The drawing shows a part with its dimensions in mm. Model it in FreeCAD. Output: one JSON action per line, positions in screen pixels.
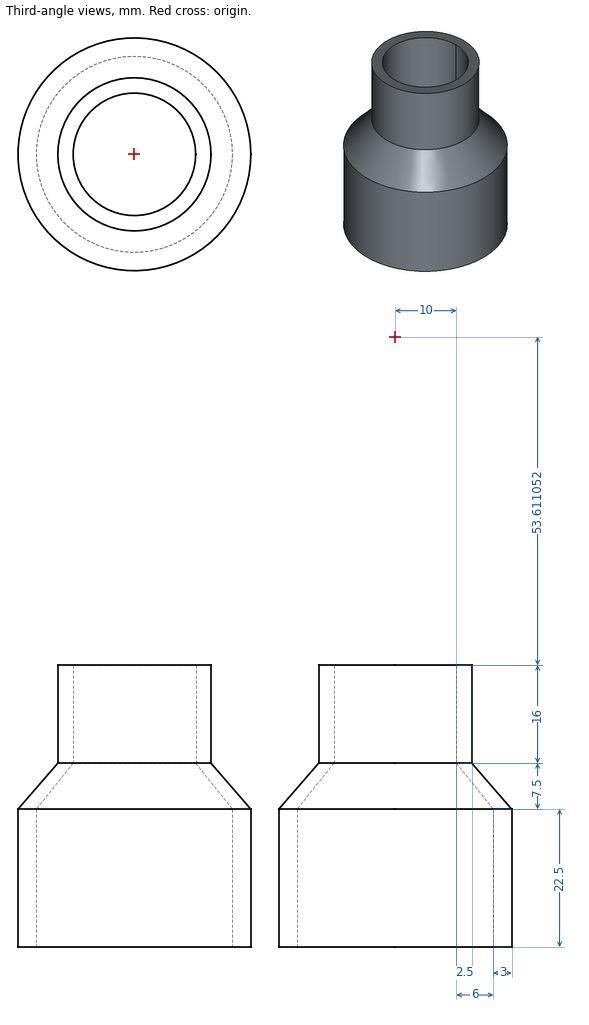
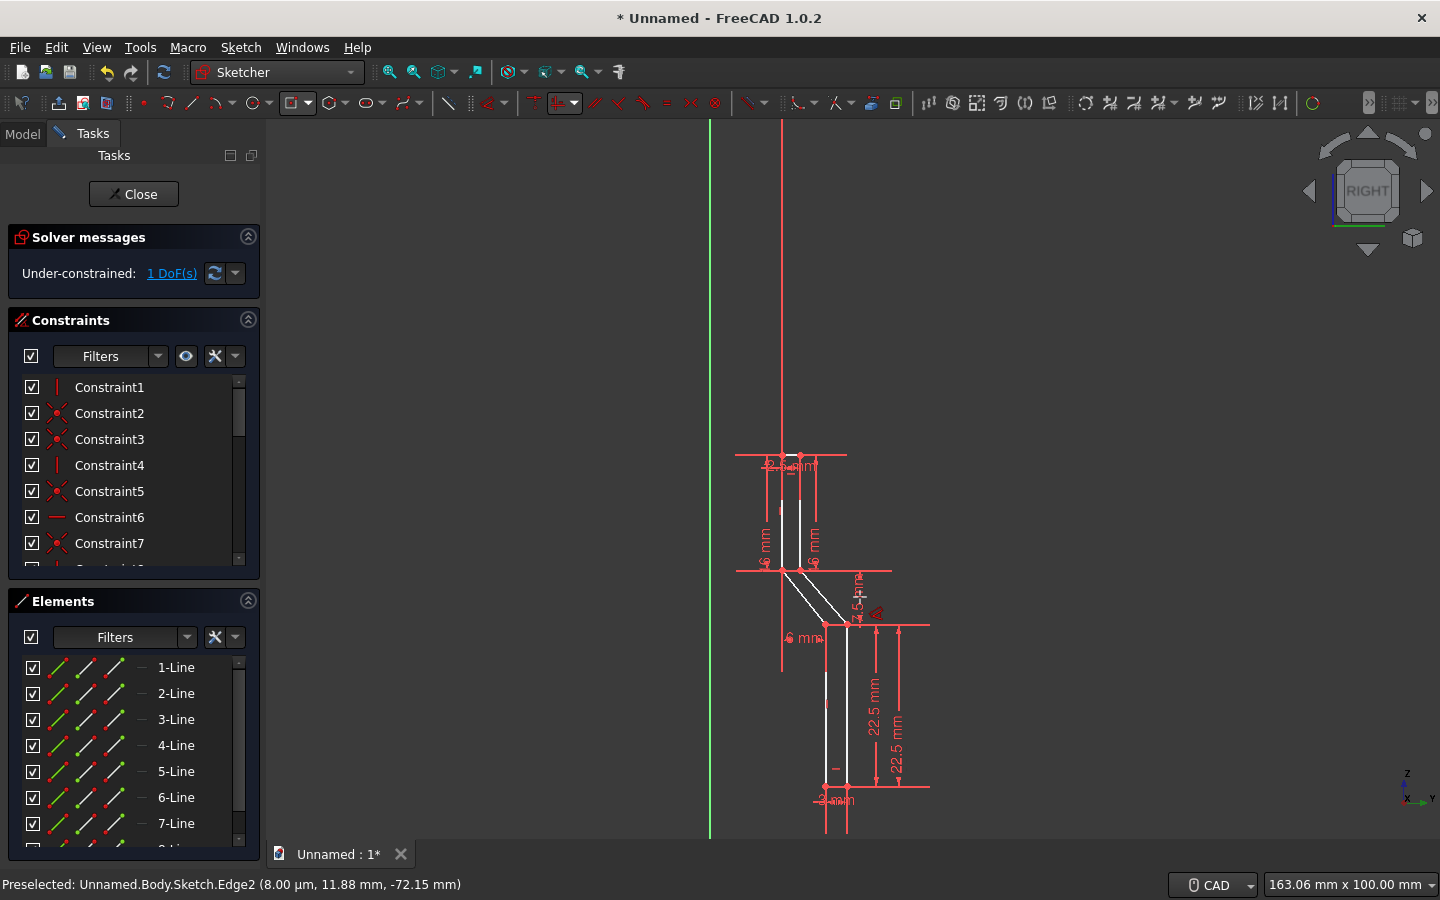
{"action": "left_click", "coordinate": [782, 455]}
{"action": "left_click", "coordinate": [676, 301]}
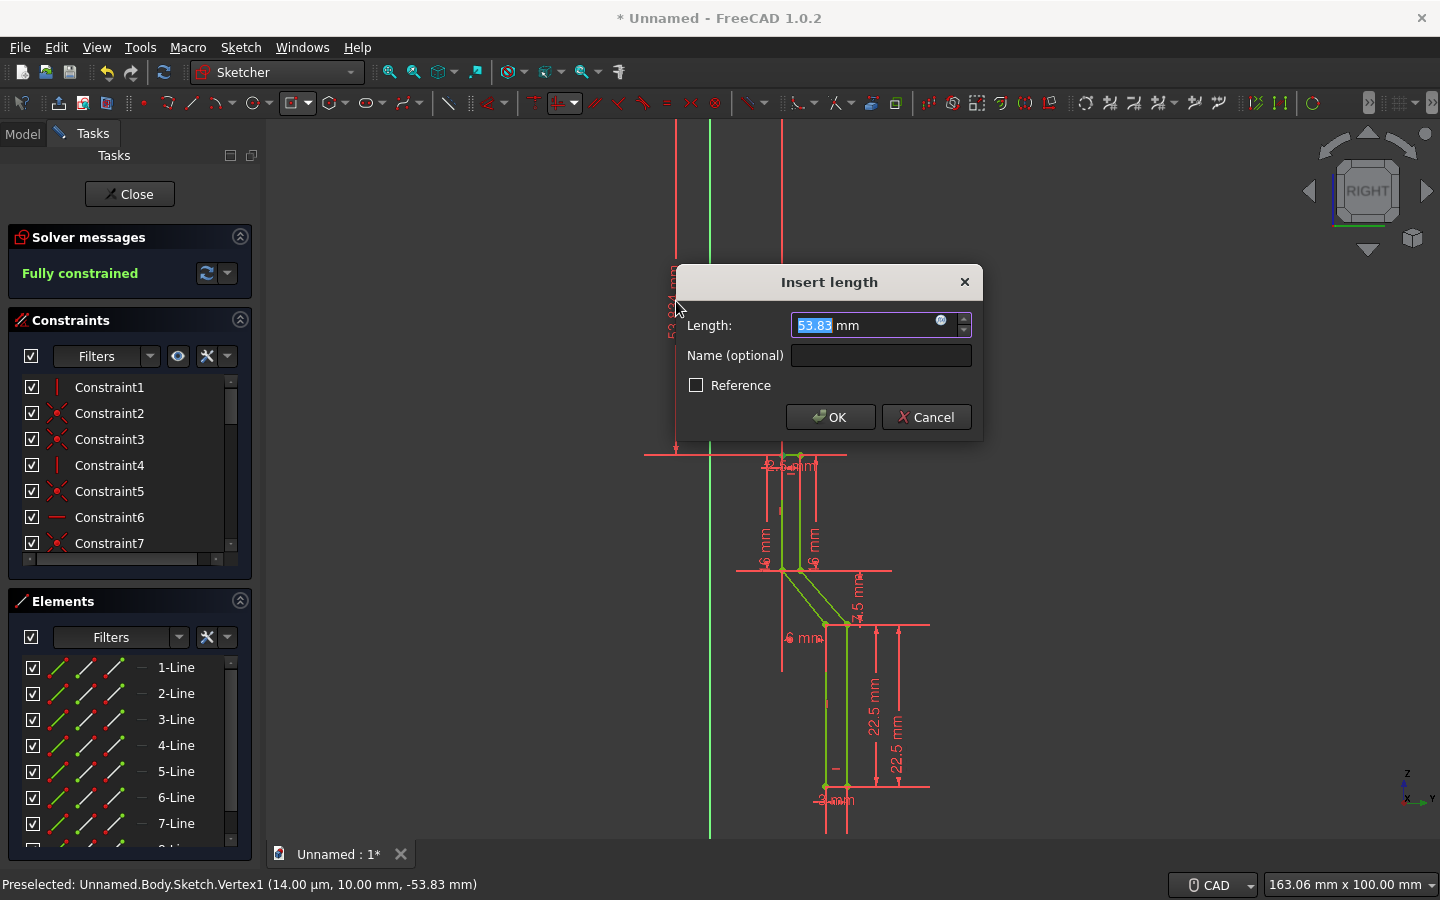
{"action": "type", "text": "53.611052"}
{"action": "key", "text": "Return"}
{"action": "key", "text": "Escape"}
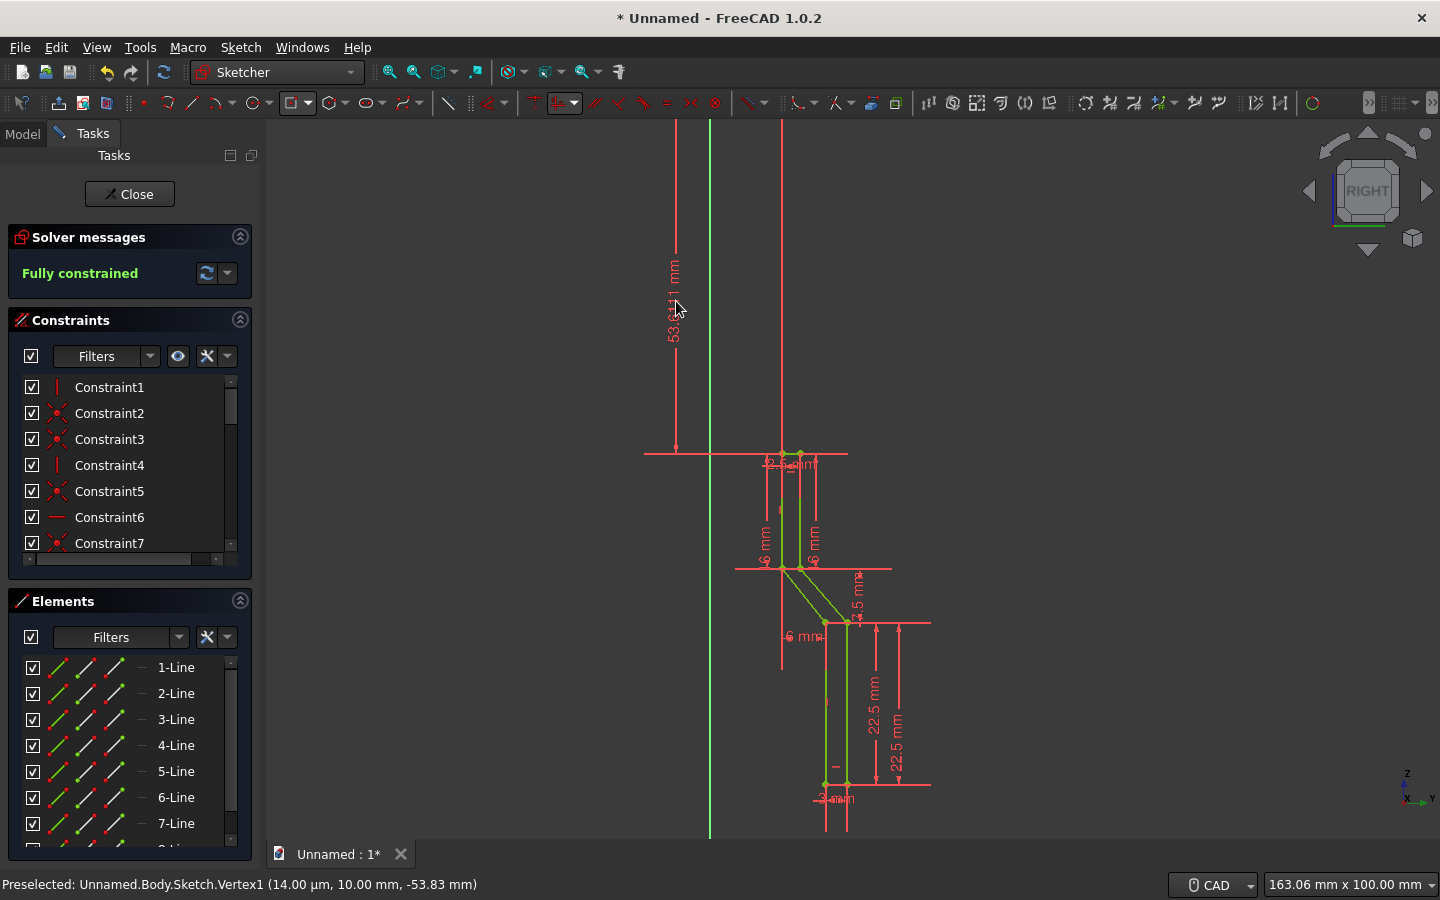
{"action": "left_click", "coordinate": [130, 194]}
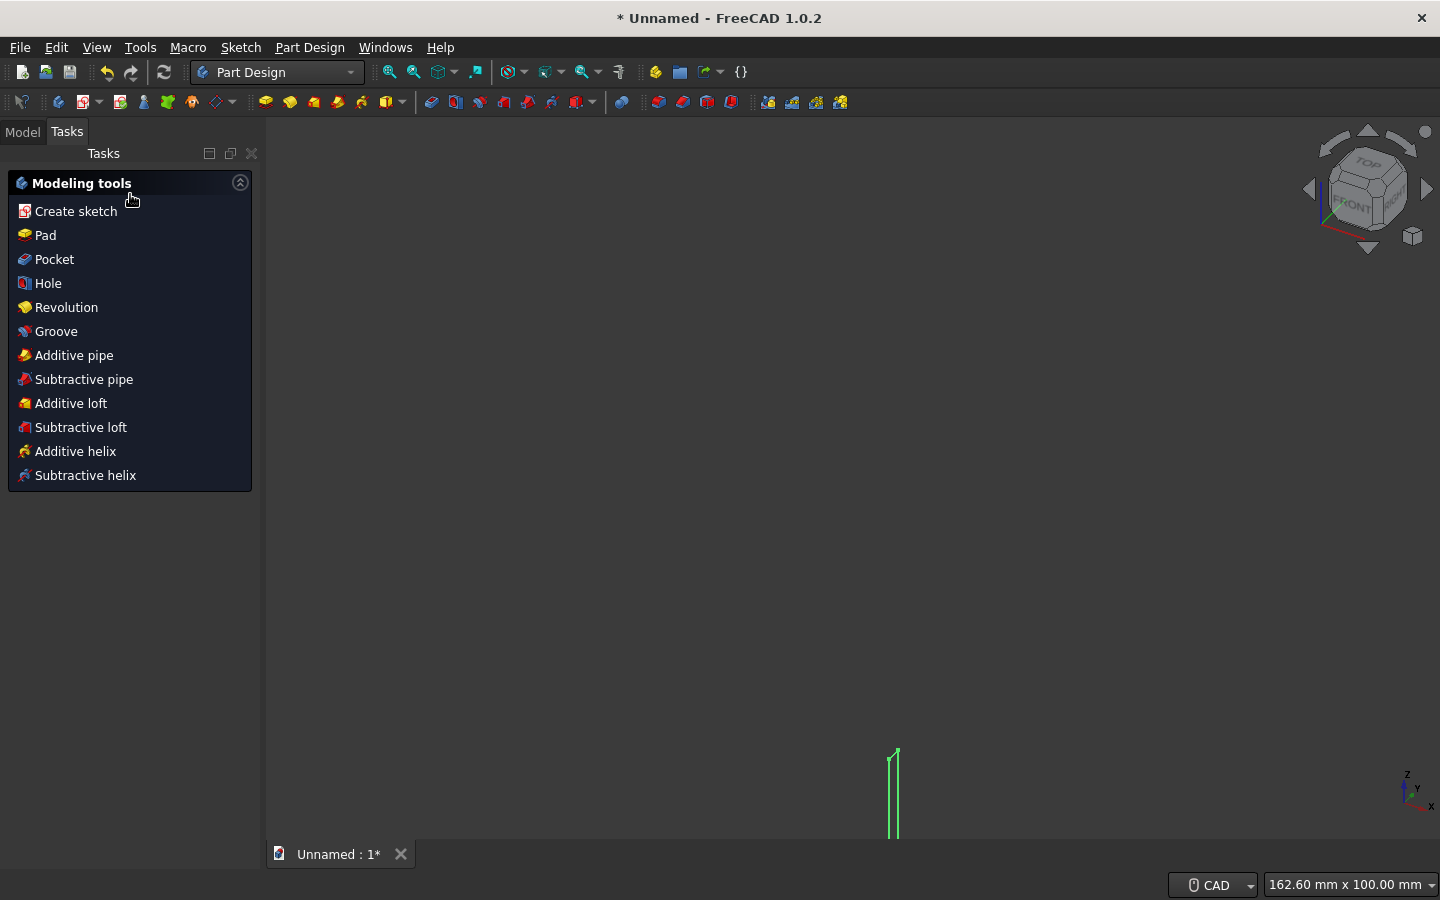
{"action": "left_click", "coordinate": [290, 102]}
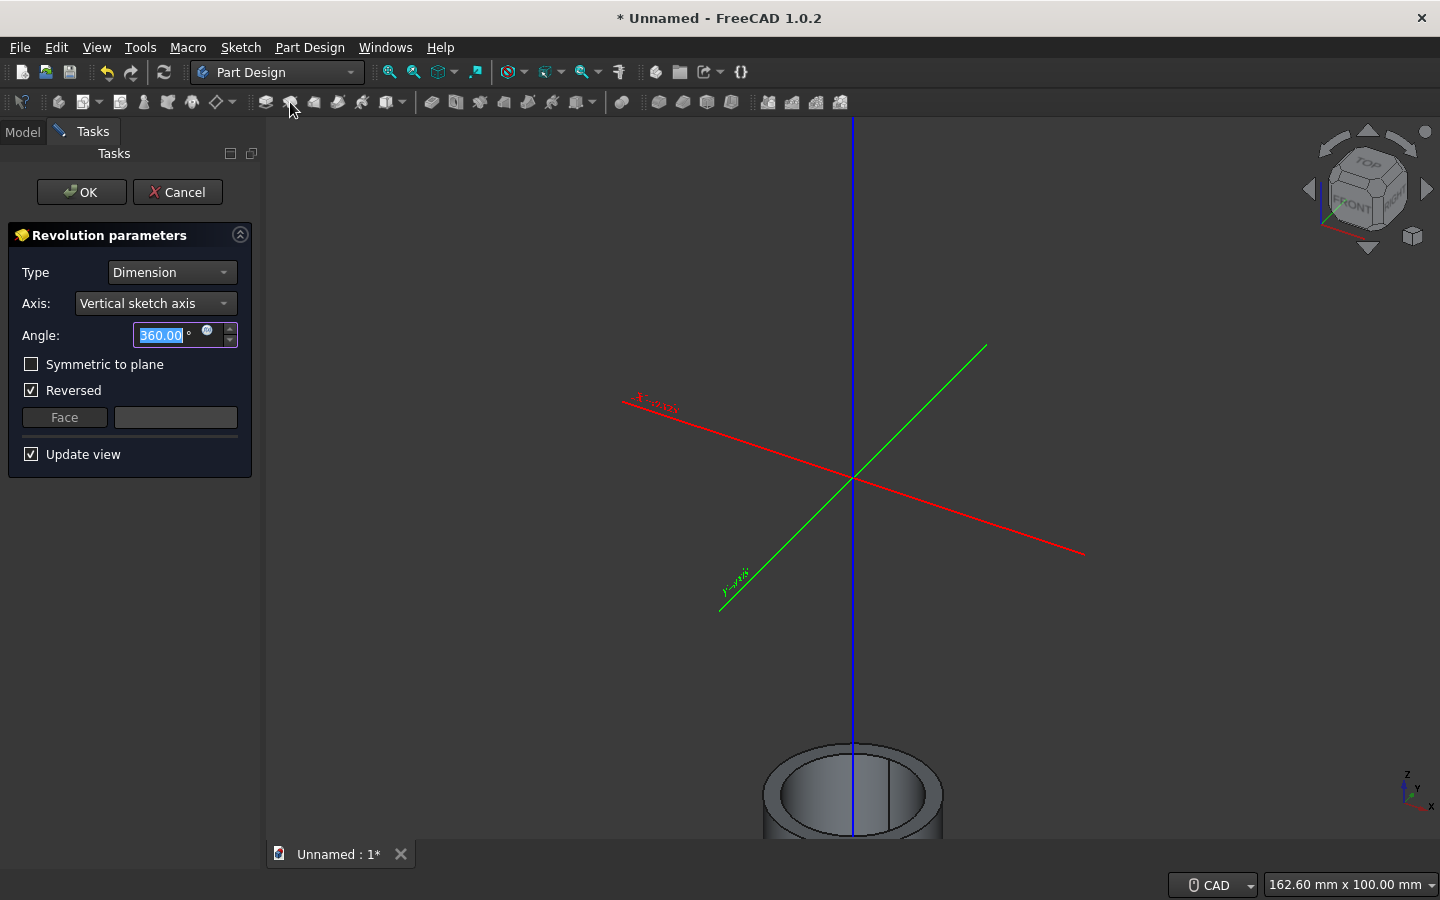
{"action": "left_click", "coordinate": [82, 192]}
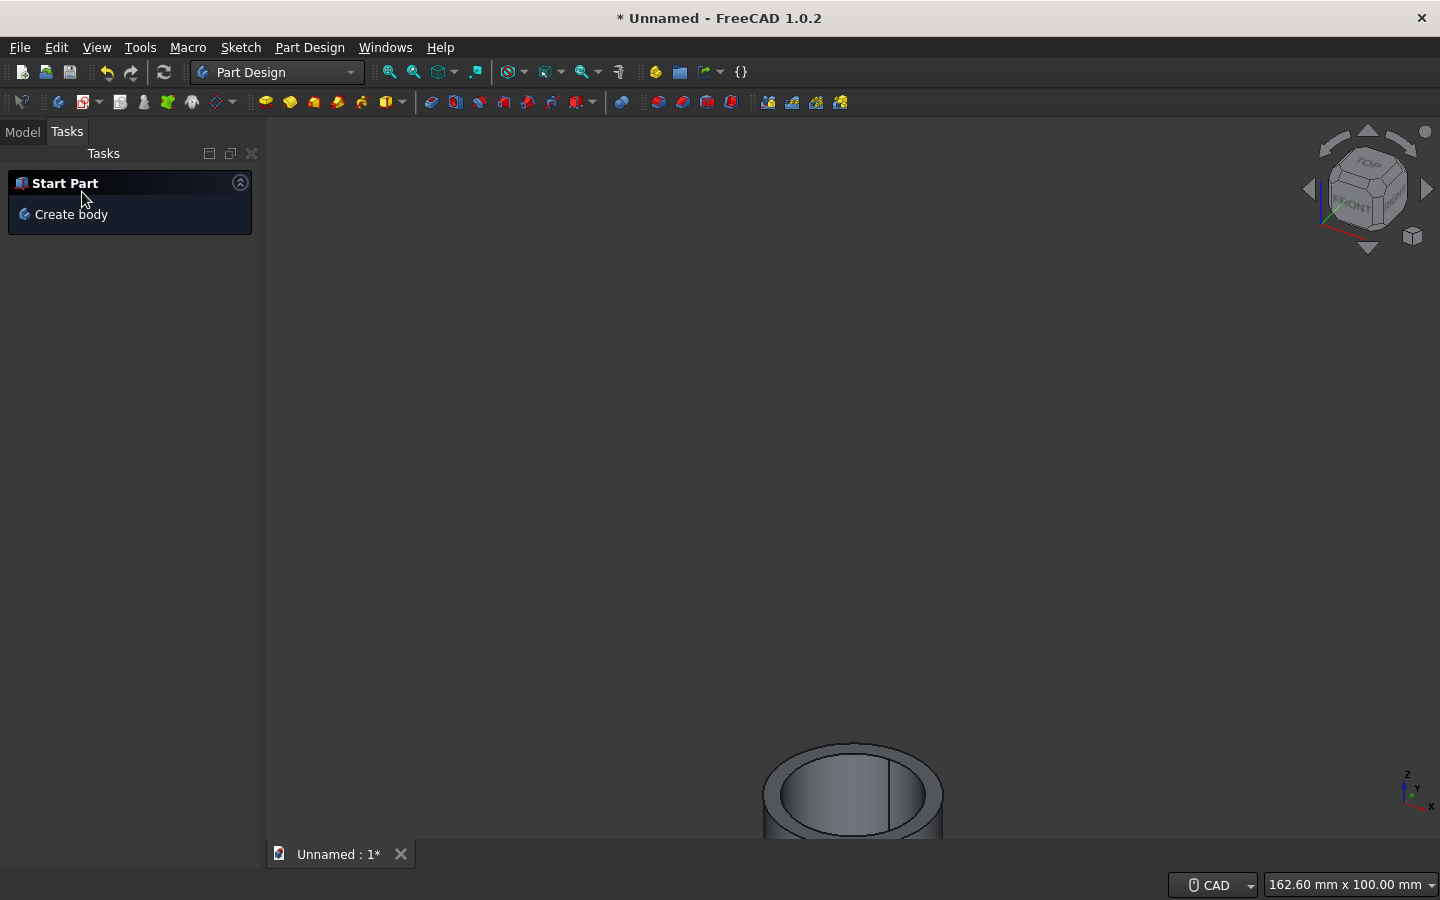
{"action": "key", "text": "0"}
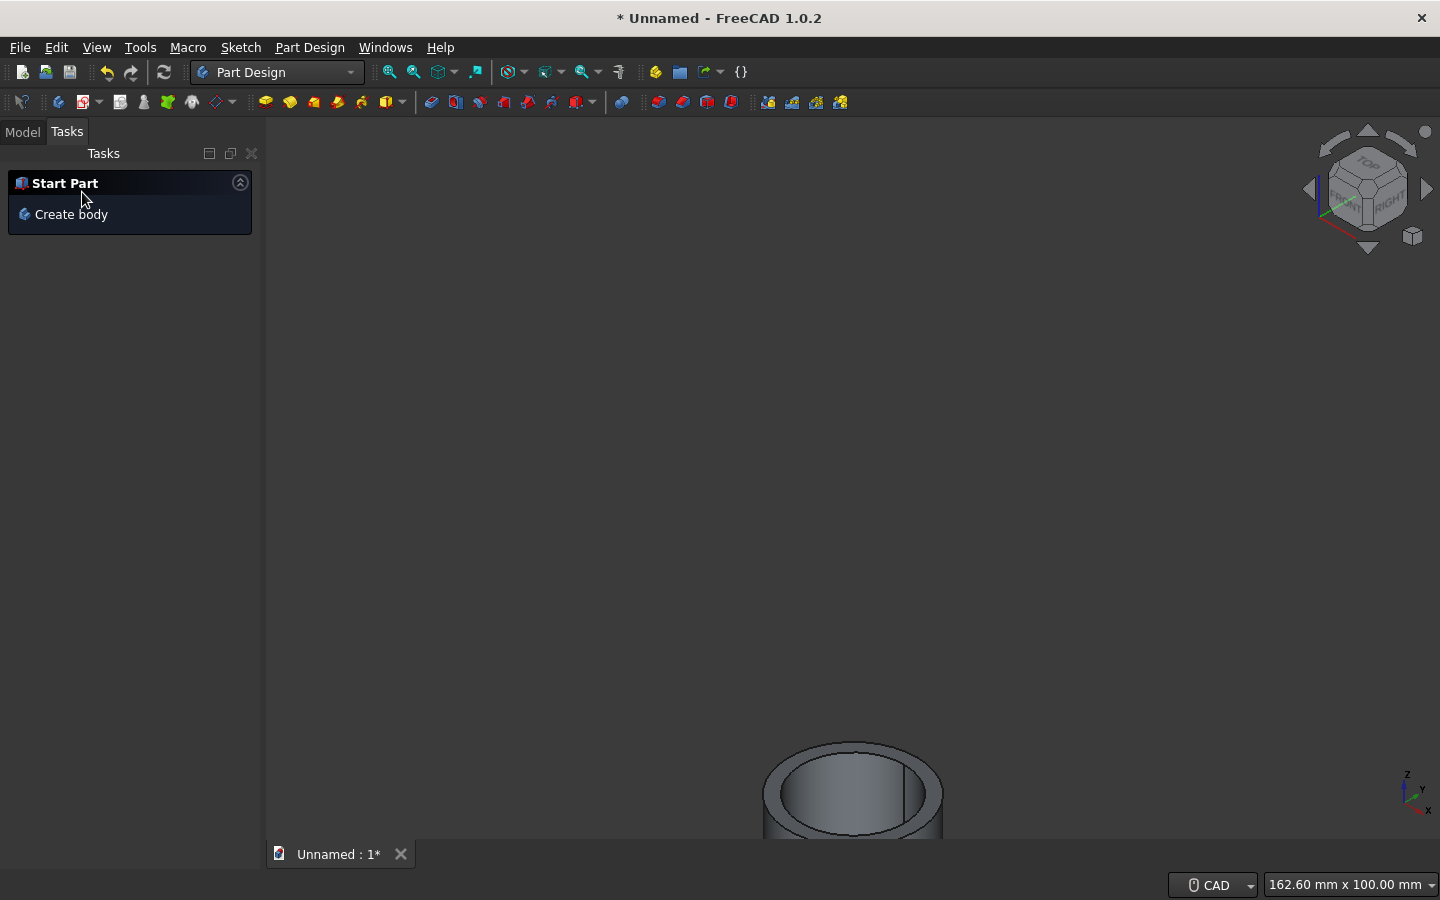
{"action": "left_click", "coordinate": [390, 72]}